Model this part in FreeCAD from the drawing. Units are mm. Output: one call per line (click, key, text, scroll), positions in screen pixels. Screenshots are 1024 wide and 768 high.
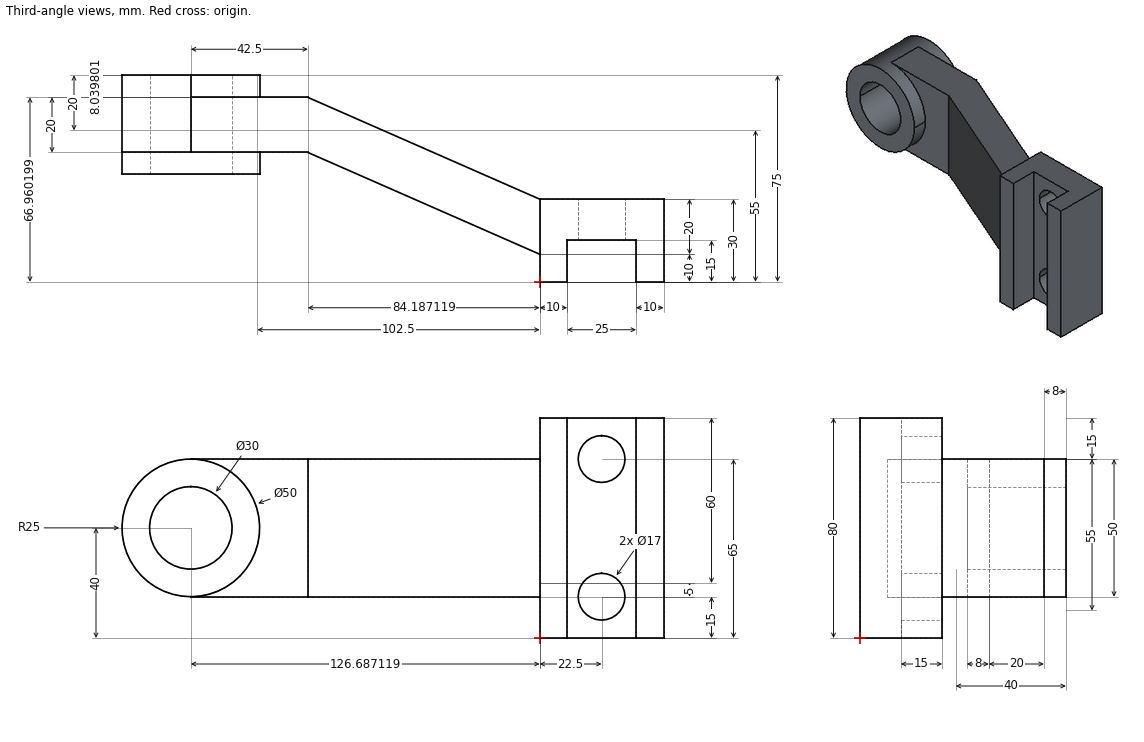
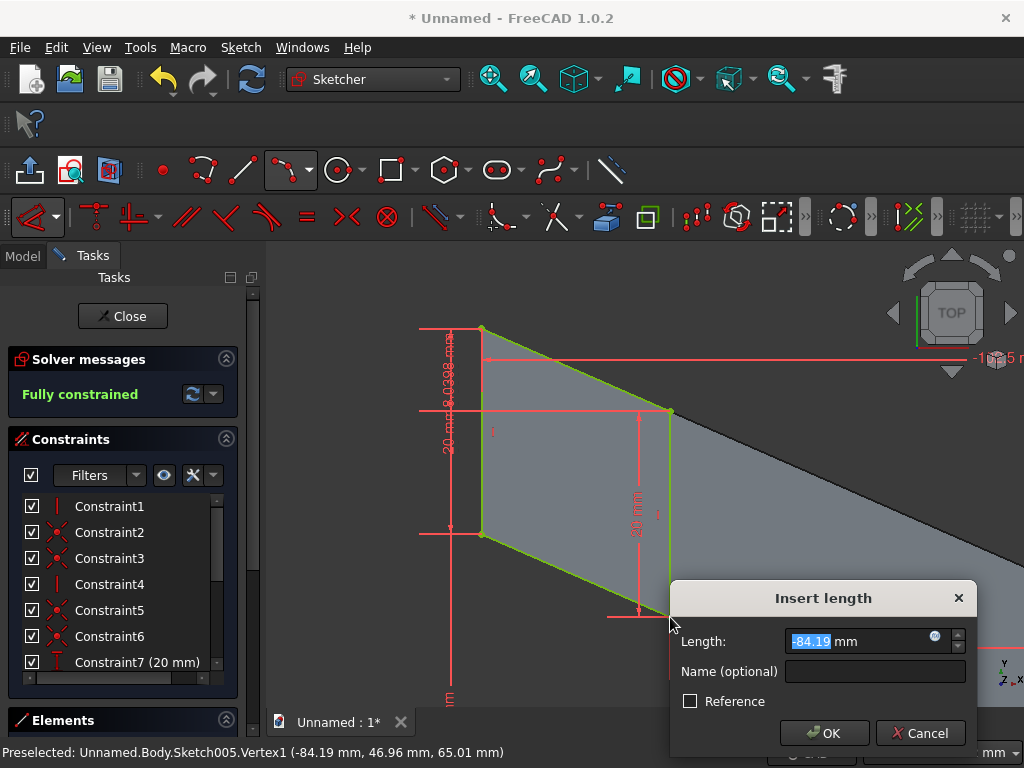
text(-84.187119)
key(Return)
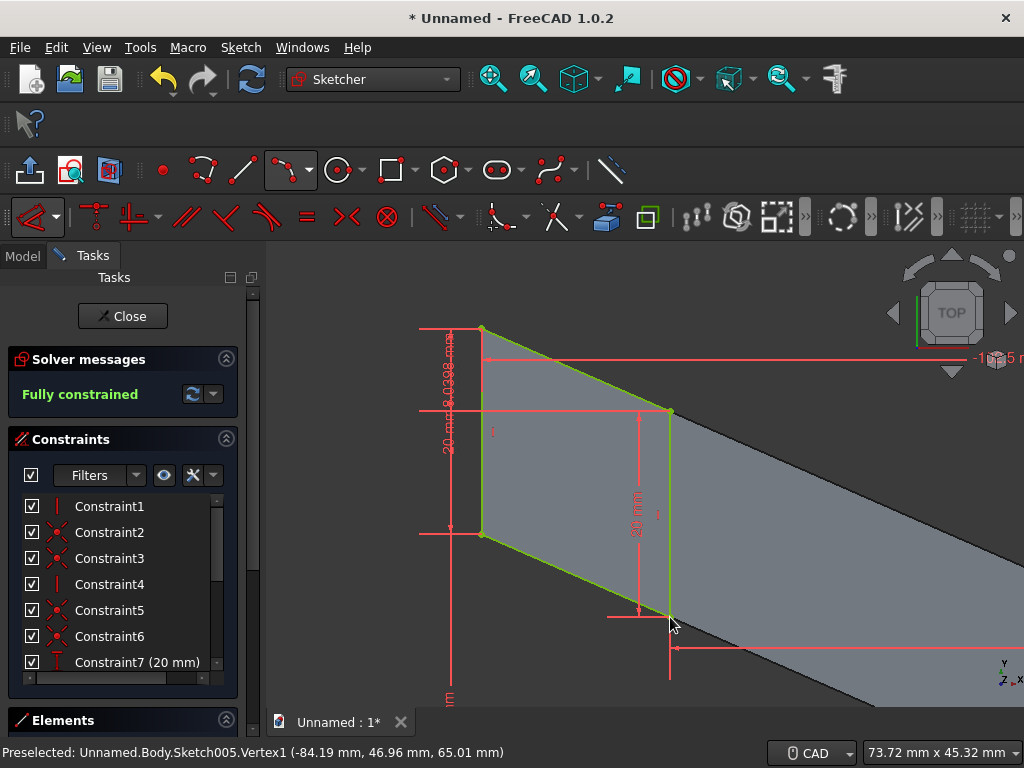
click(123, 316)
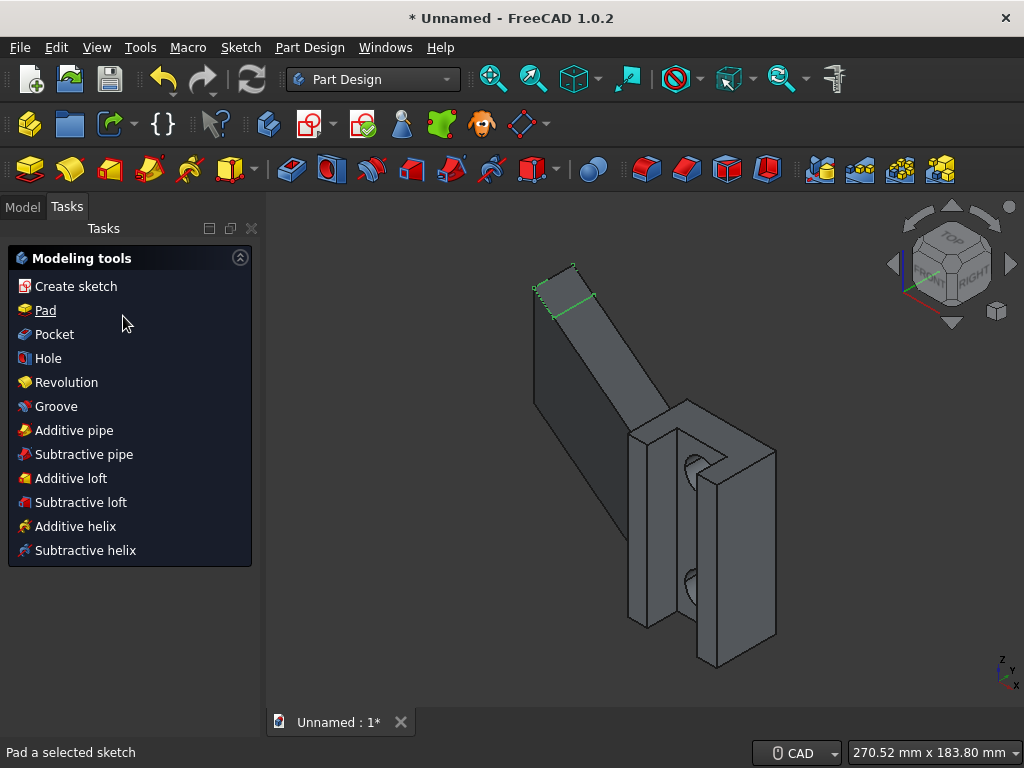
click(292, 170)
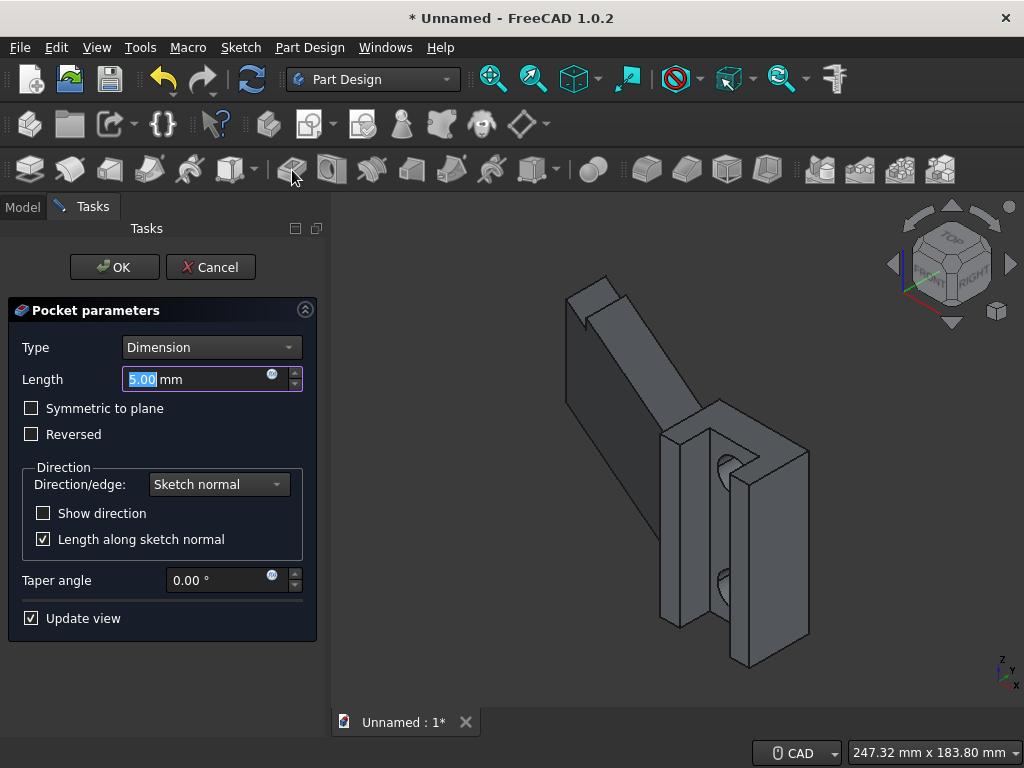
text(55)
key(Tab)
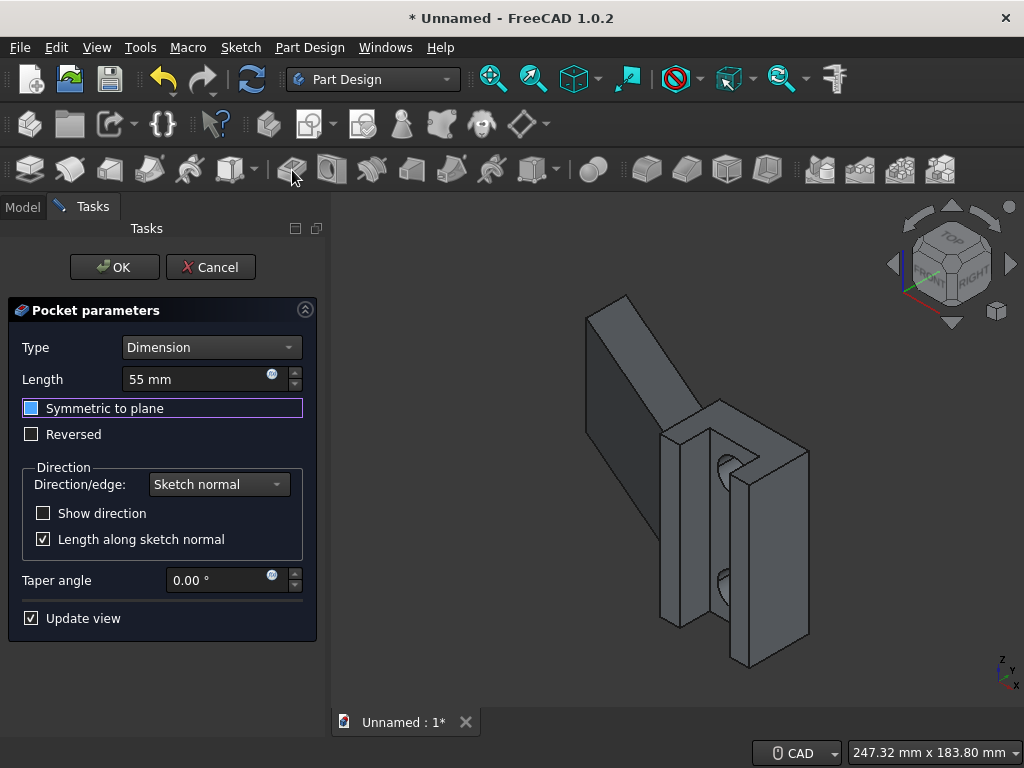
click(115, 267)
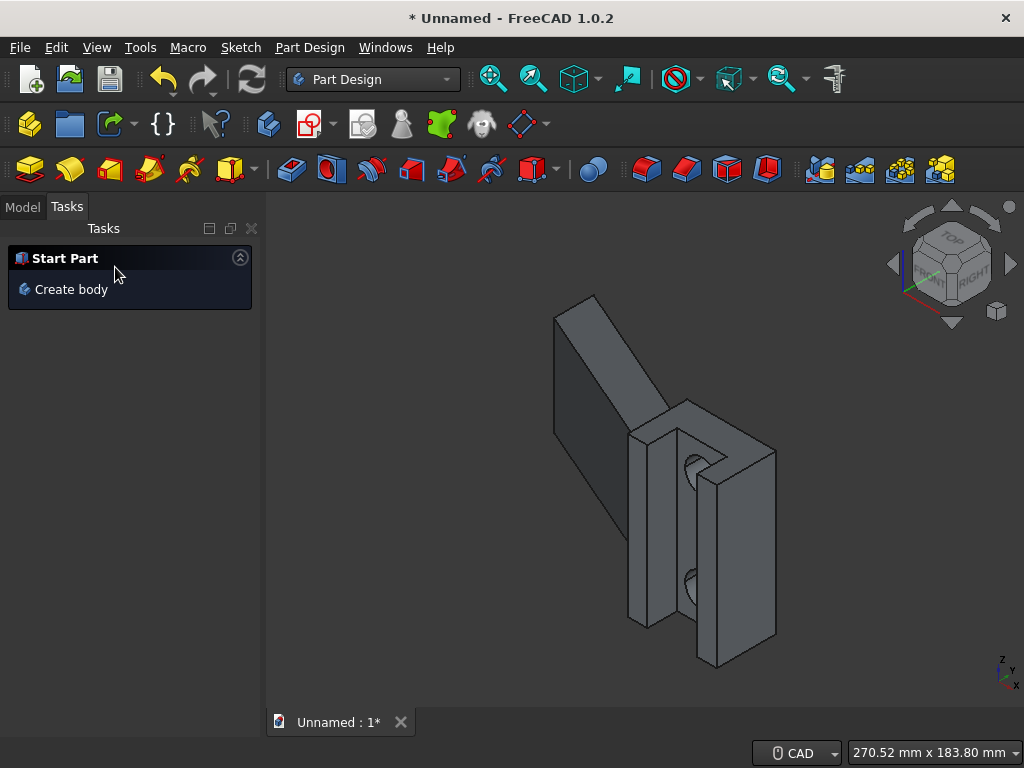
click(621, 375)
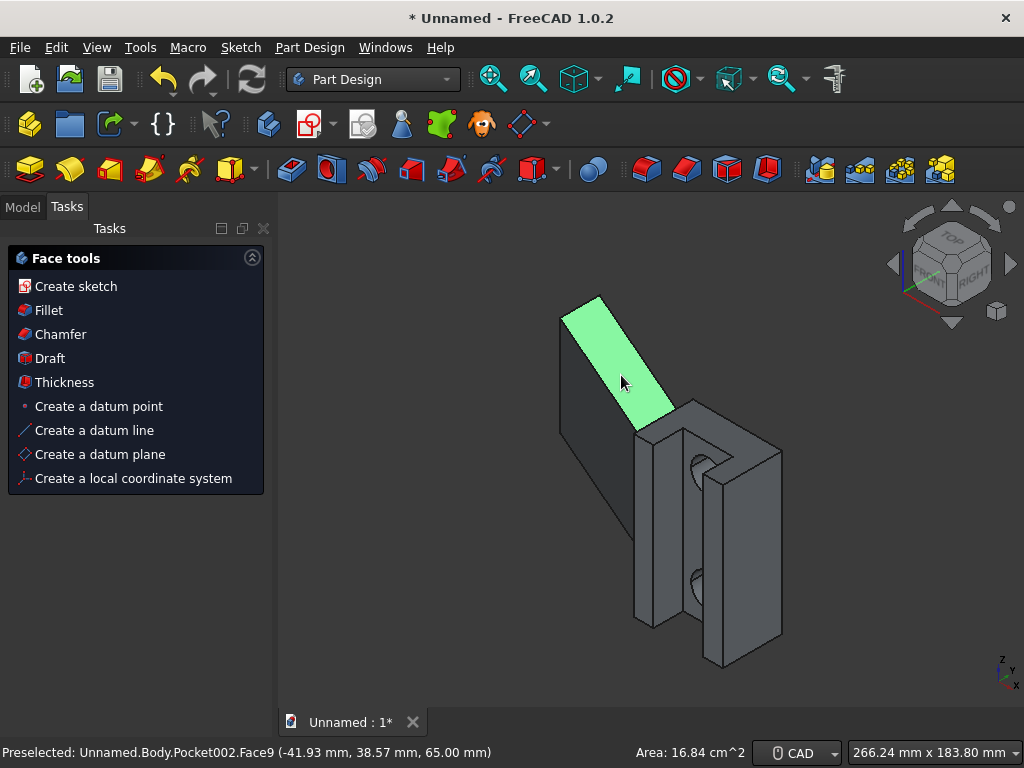
click(310, 124)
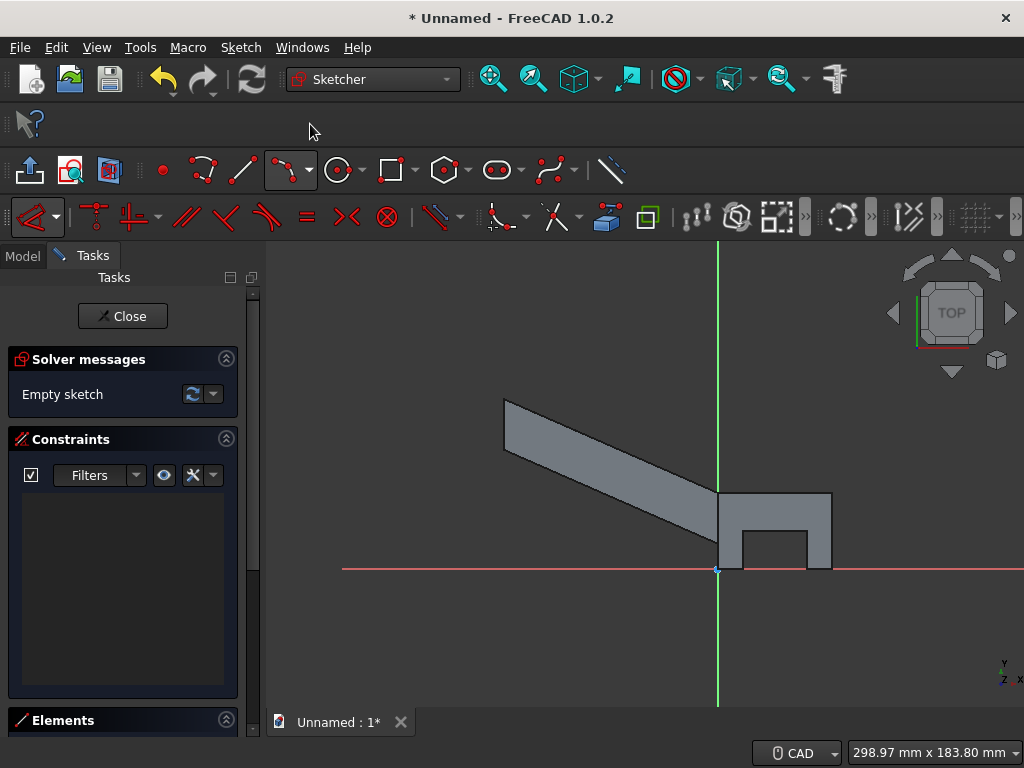
key(q)
key(s)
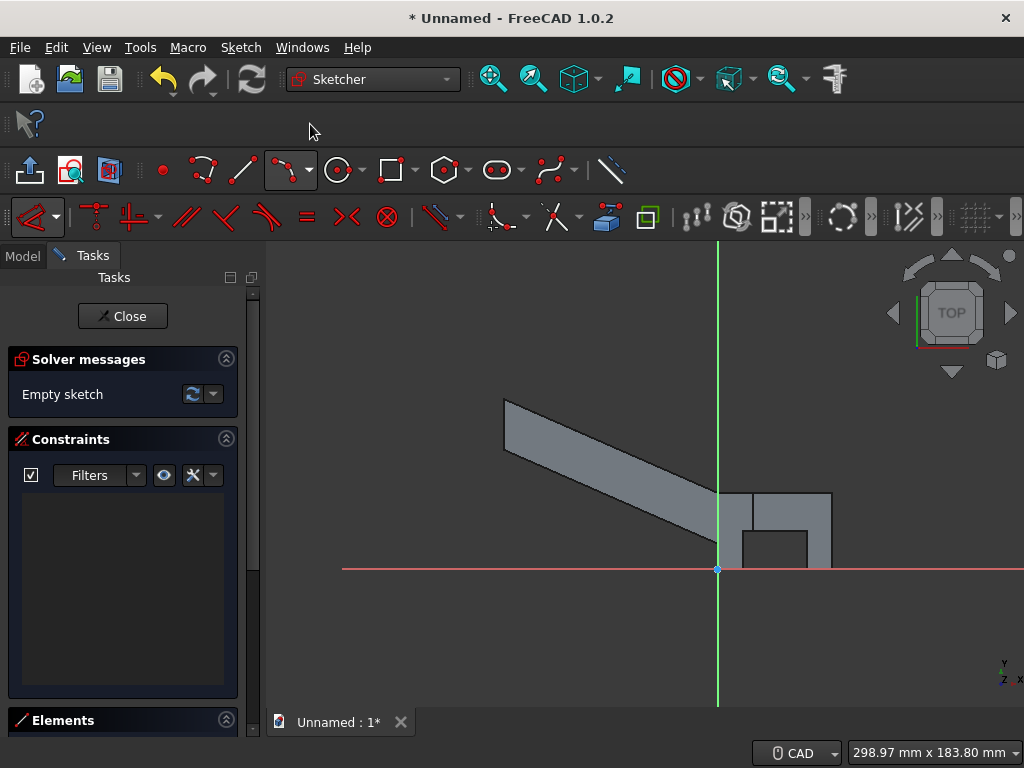
scroll(409, 409, up, 7)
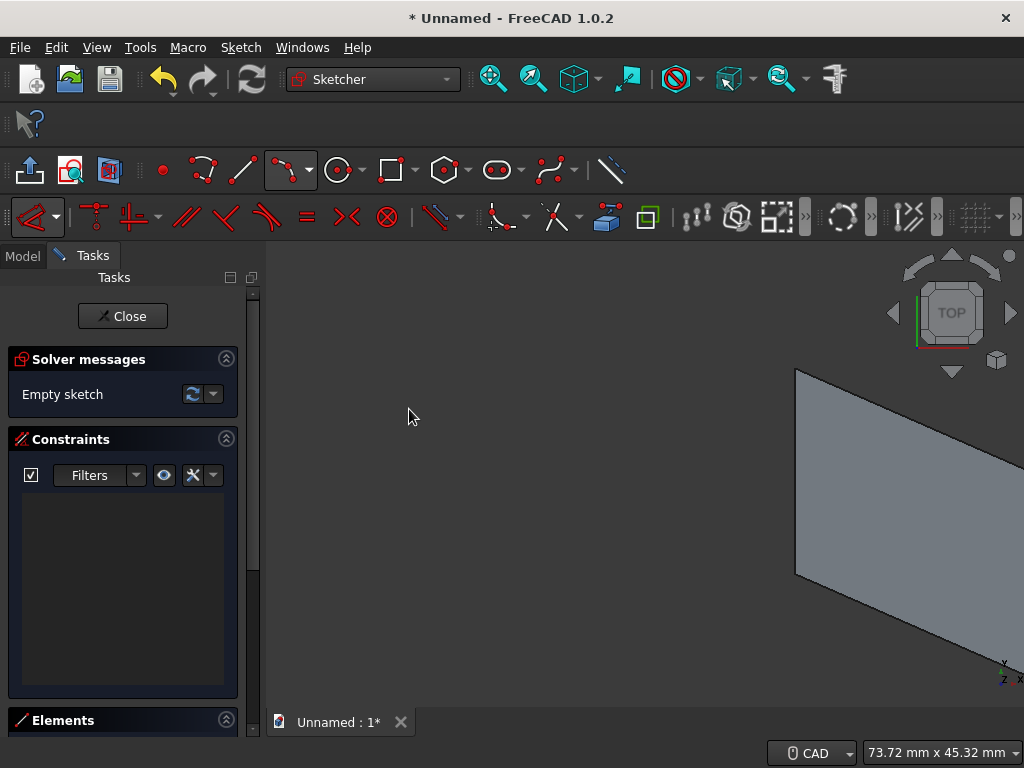
click(392, 170)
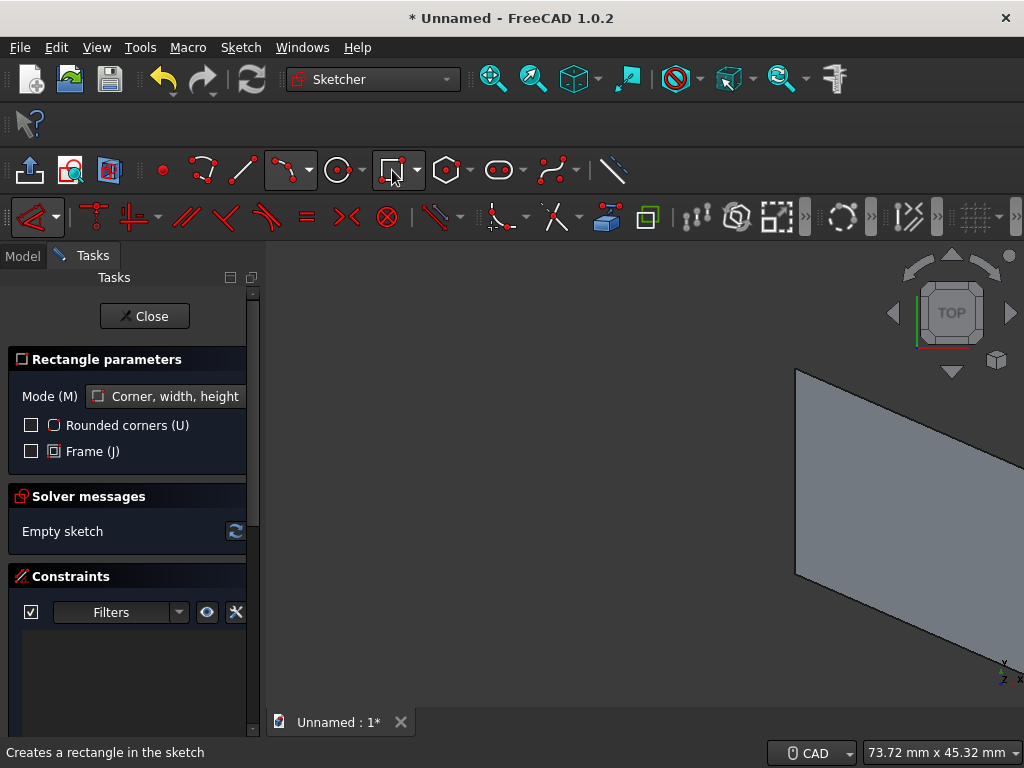
click(359, 369)
move(795, 574)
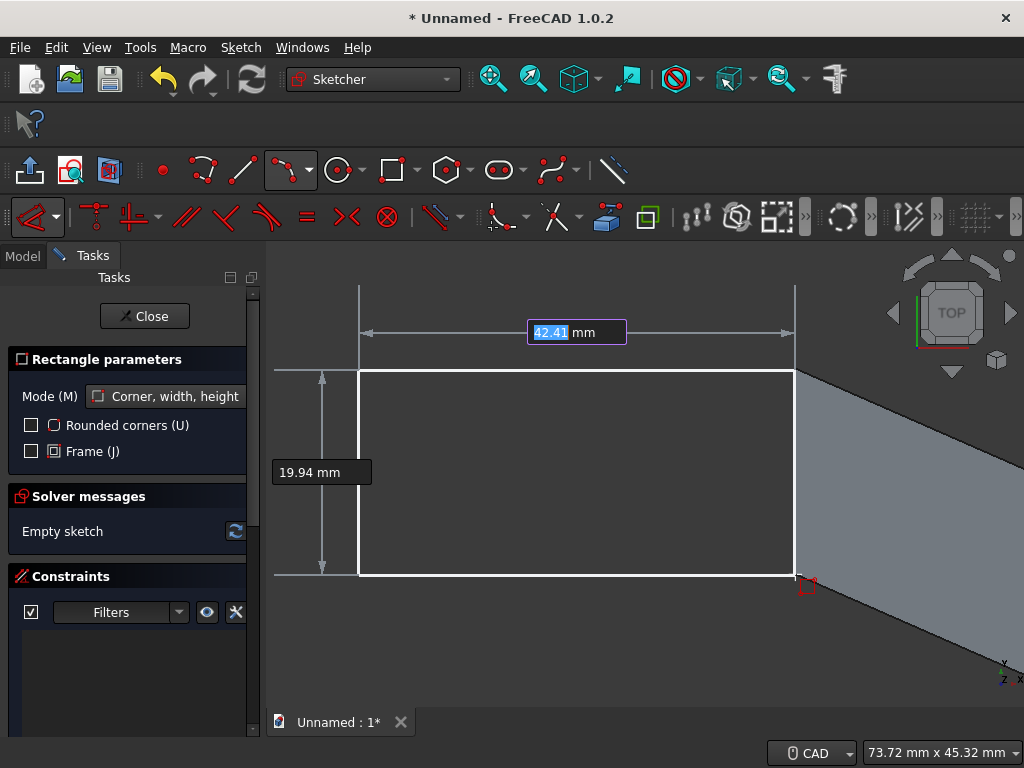
text(42.5)
key(Tab)
text(20)
key(Return)
key(Escape)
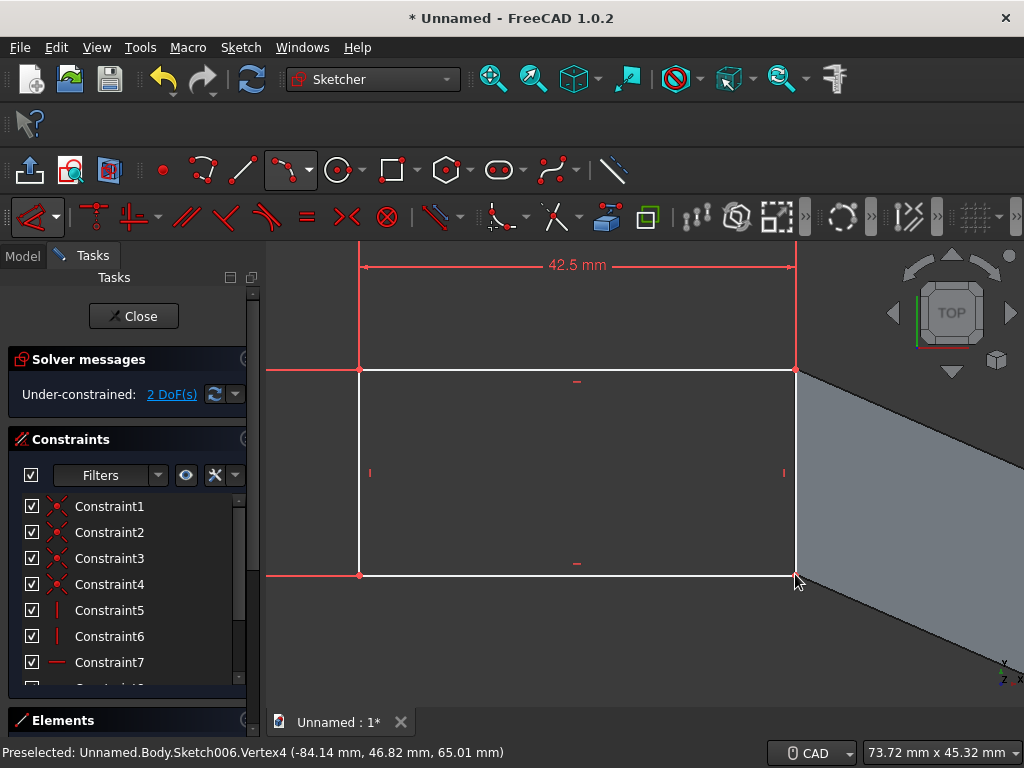
click(359, 370)